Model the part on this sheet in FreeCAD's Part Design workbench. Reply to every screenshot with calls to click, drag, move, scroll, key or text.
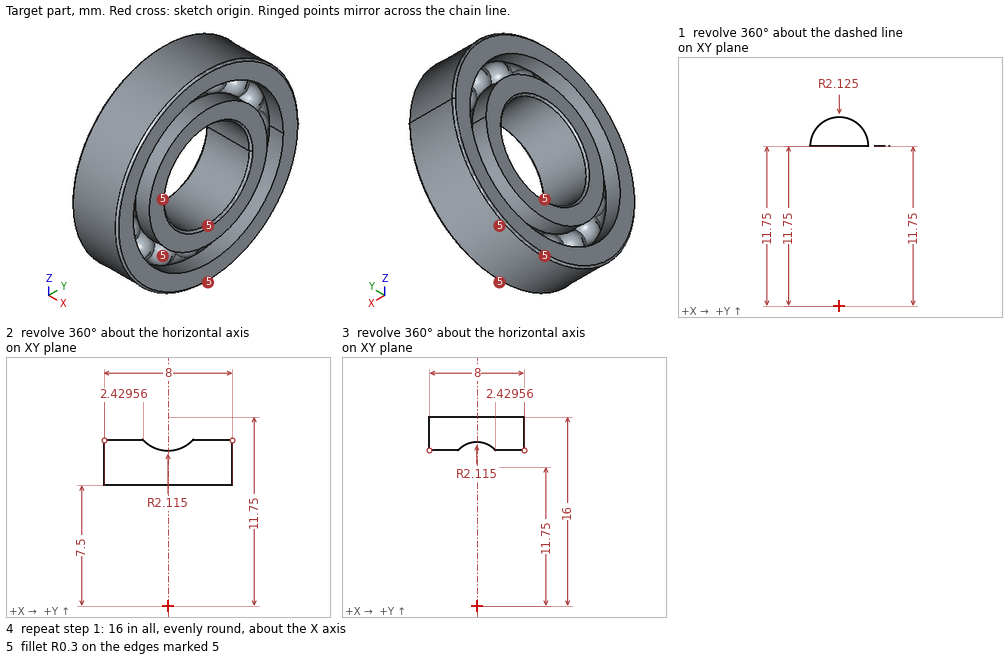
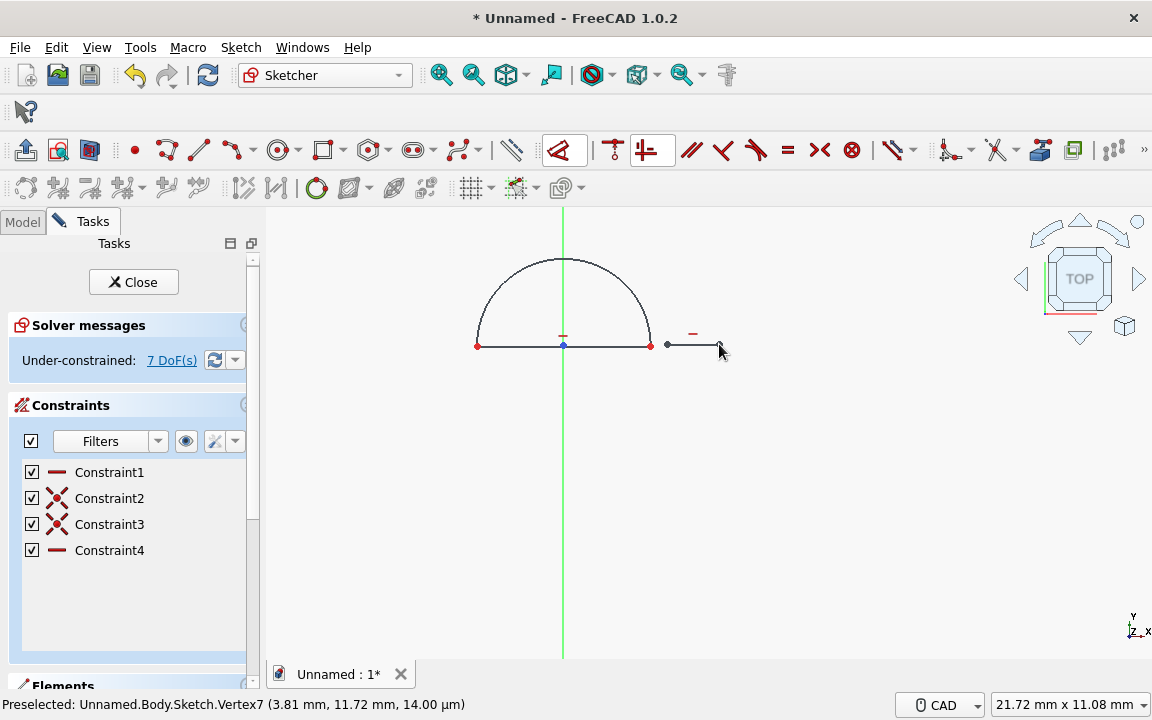
click(683, 345)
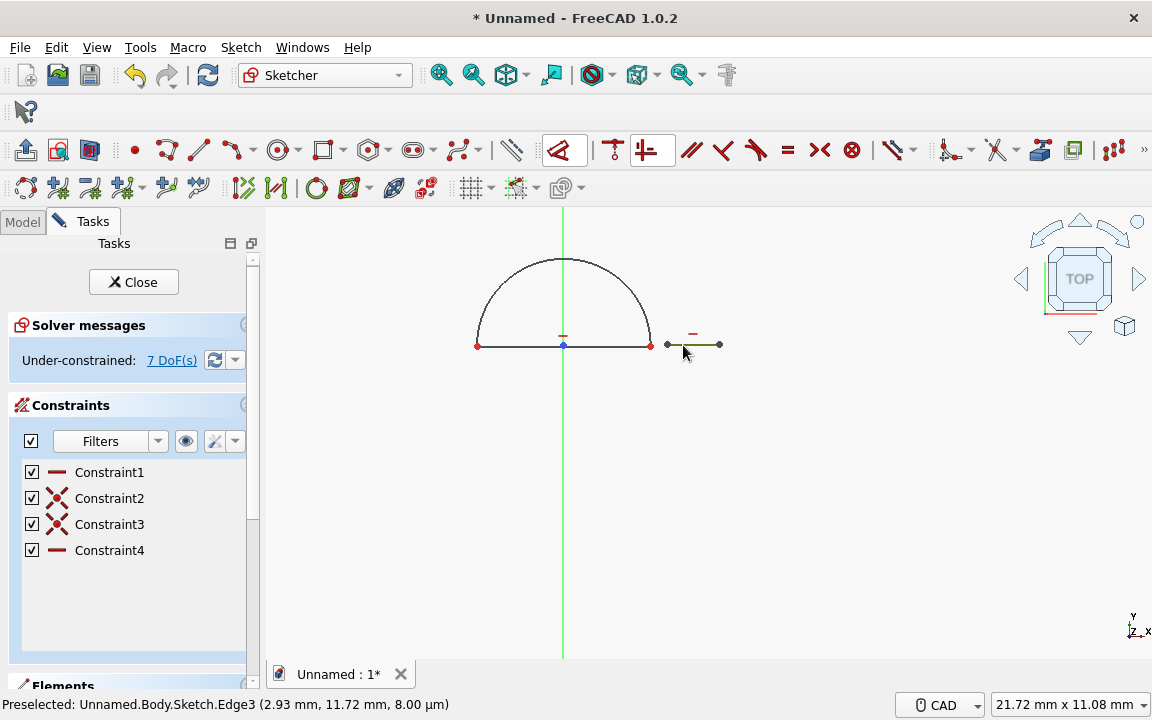
click(512, 150)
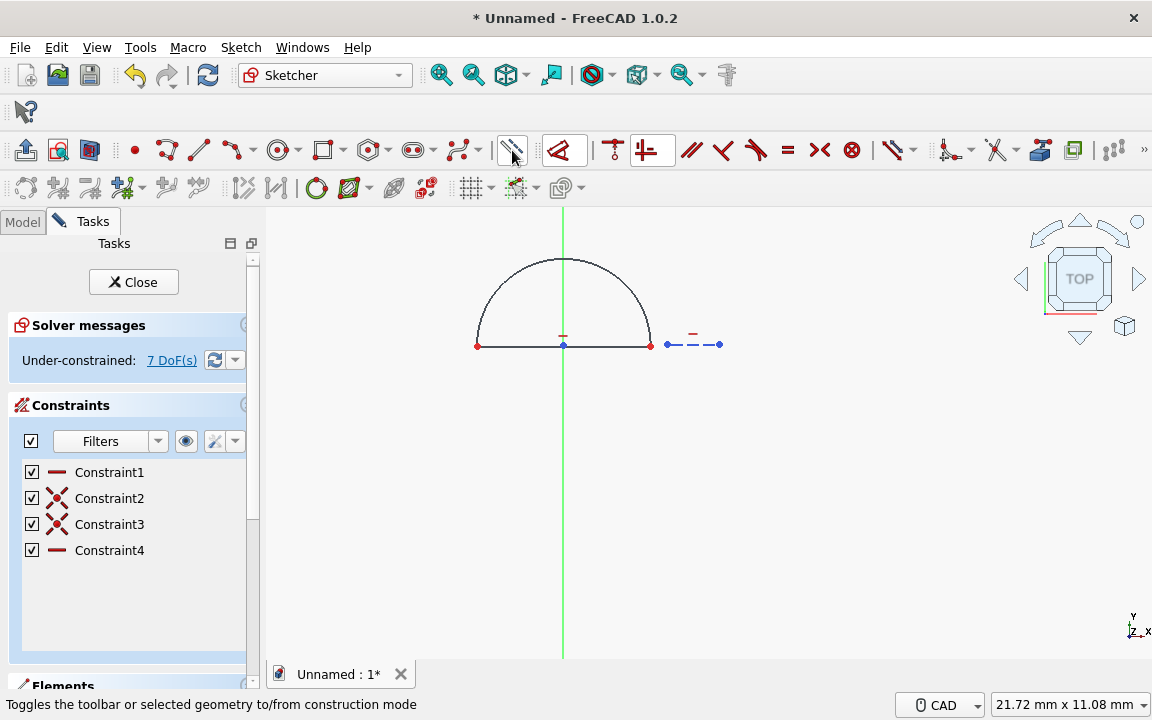
click(564, 346)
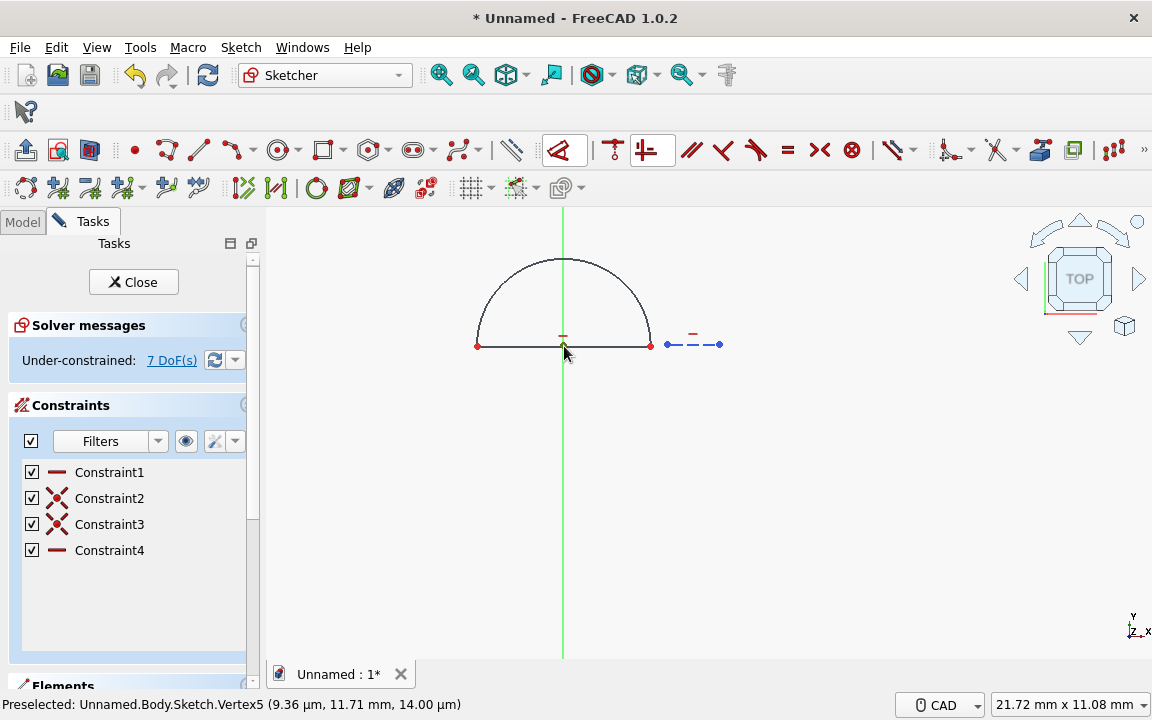
click(563, 603)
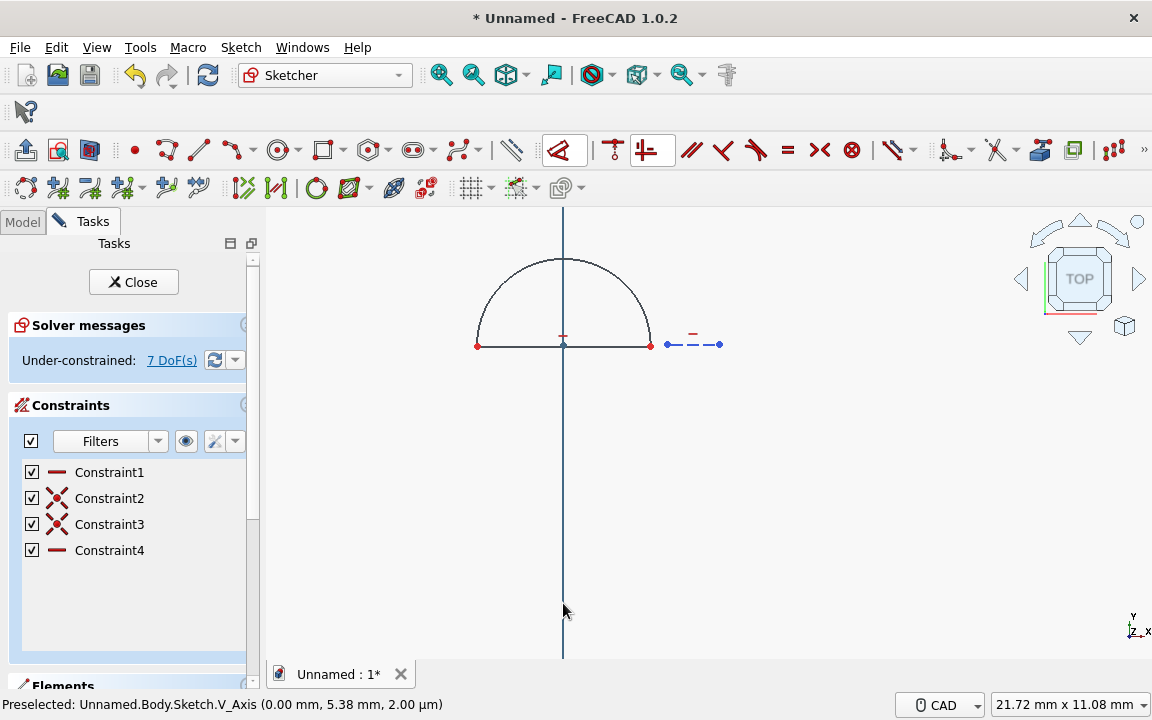
click(614, 150)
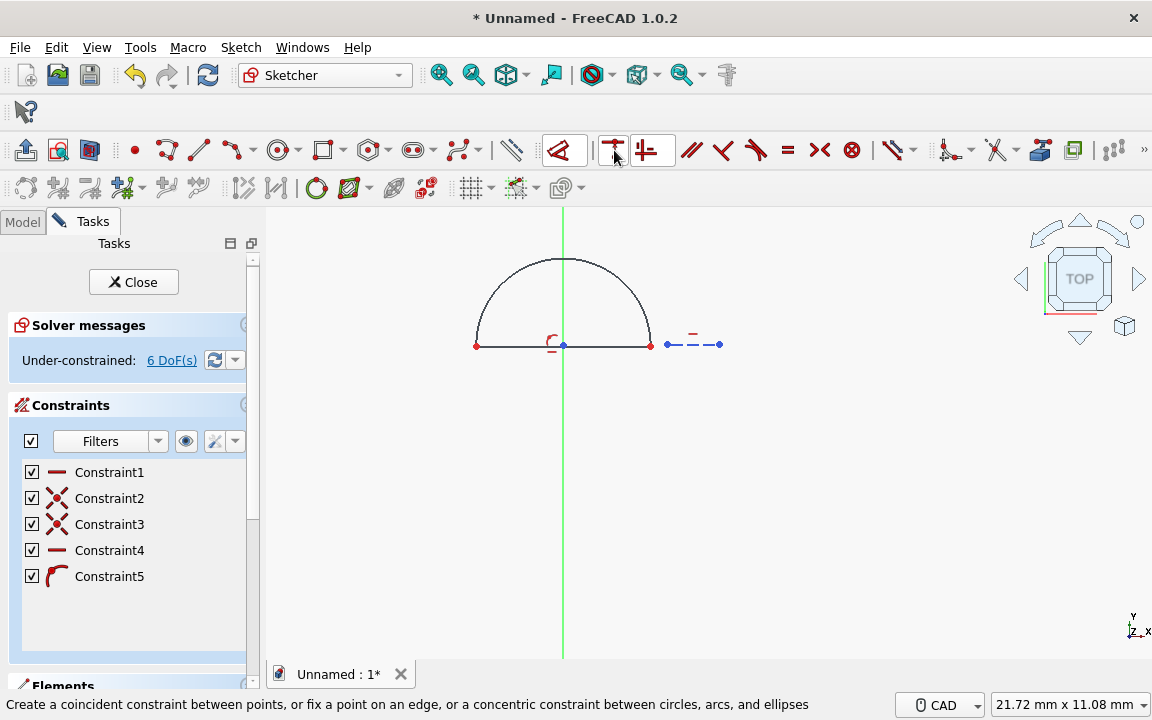
click(558, 150)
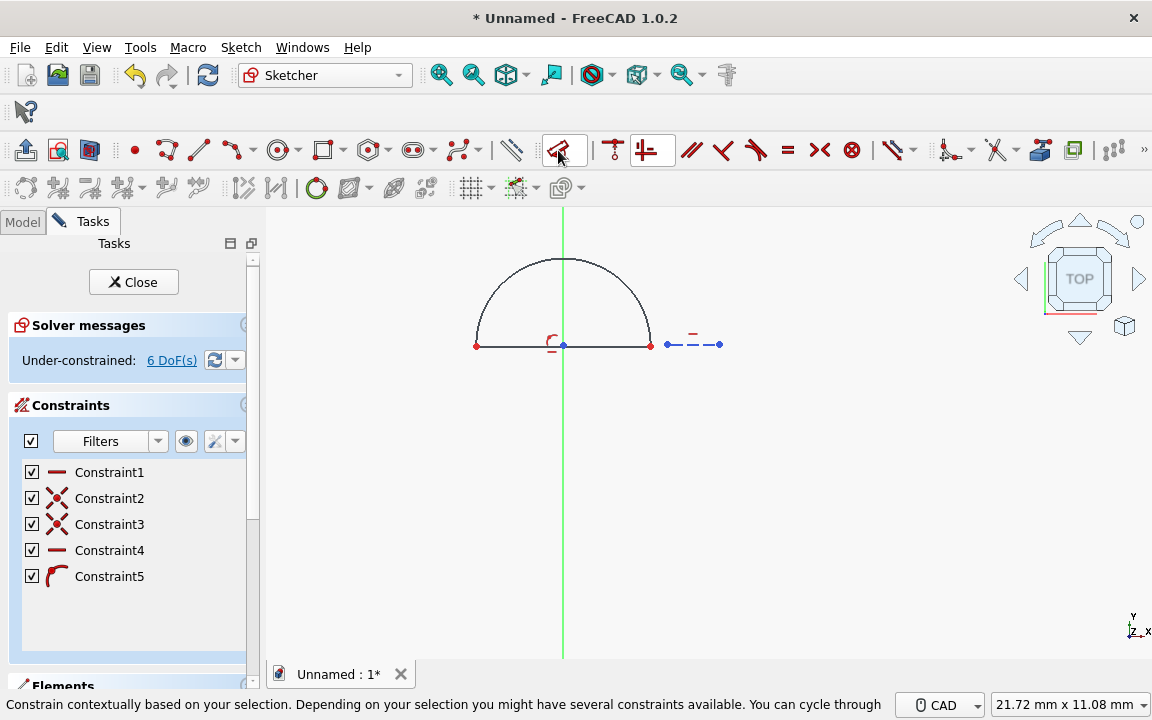
click(615, 275)
click(634, 249)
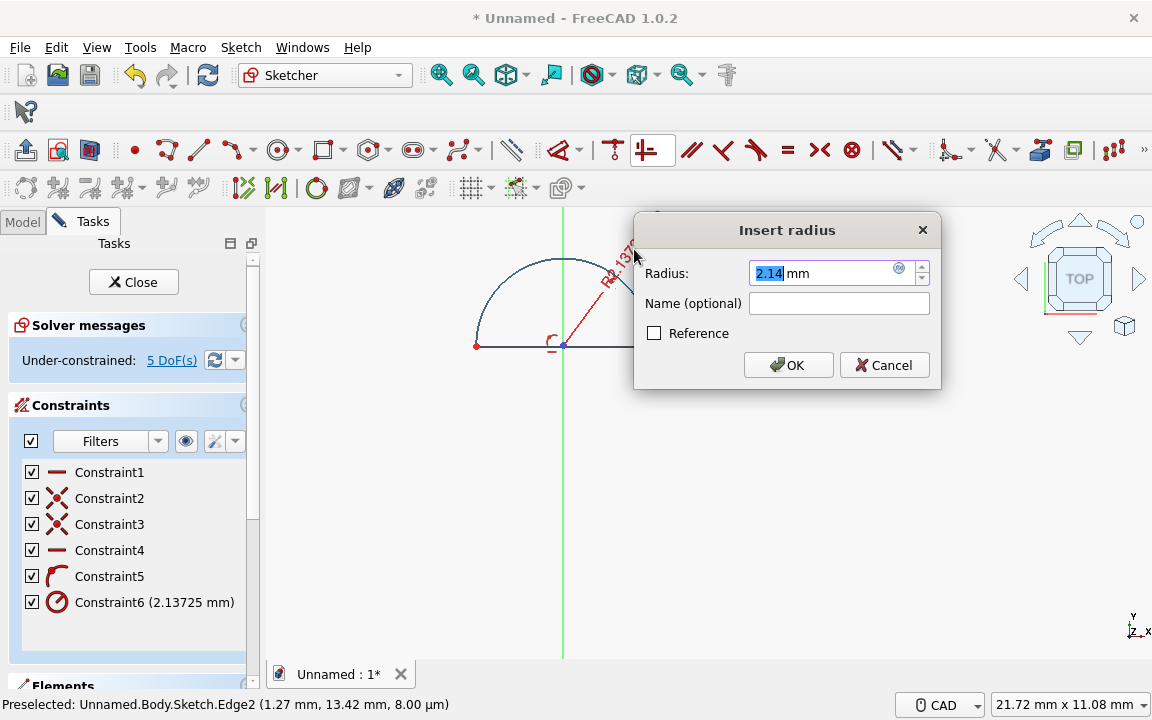
text(2.125)
key(Return)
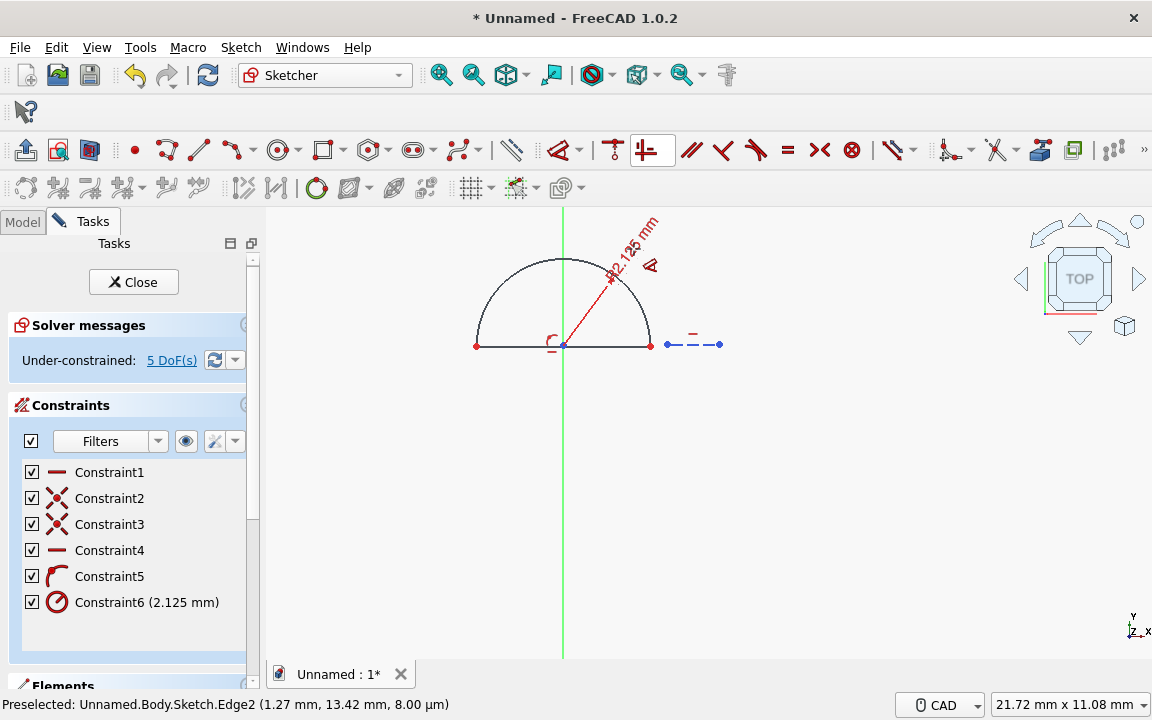
click(477, 347)
click(443, 489)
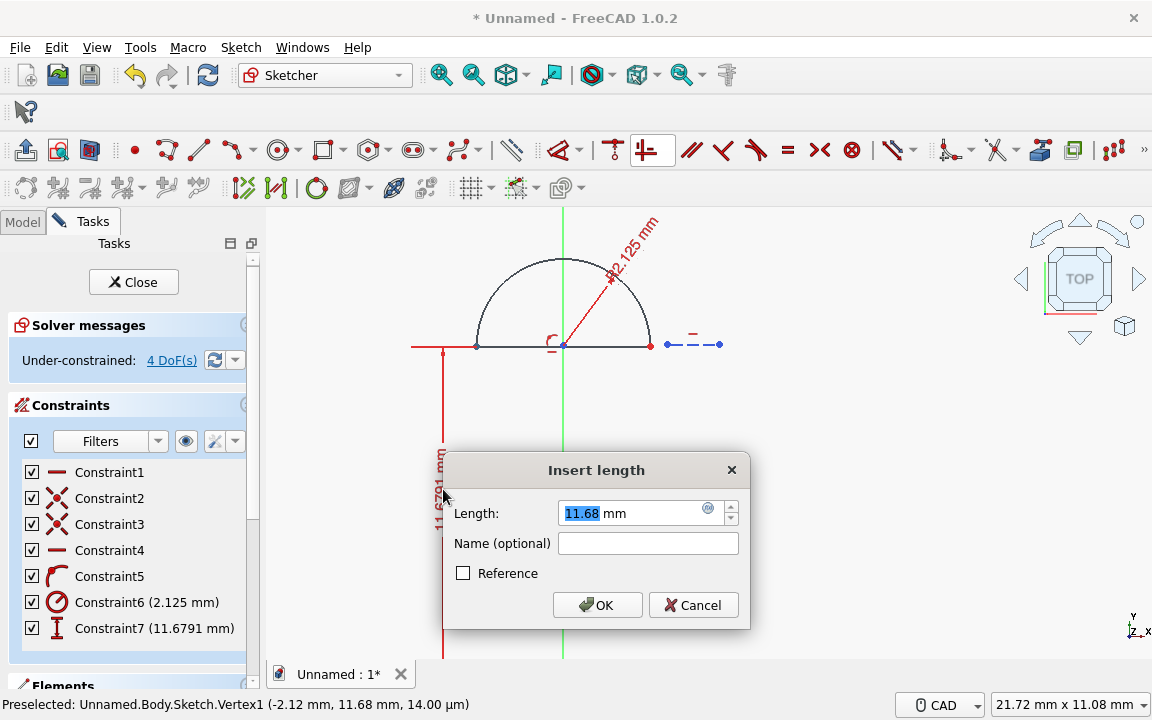
text(11.75)
key(Return)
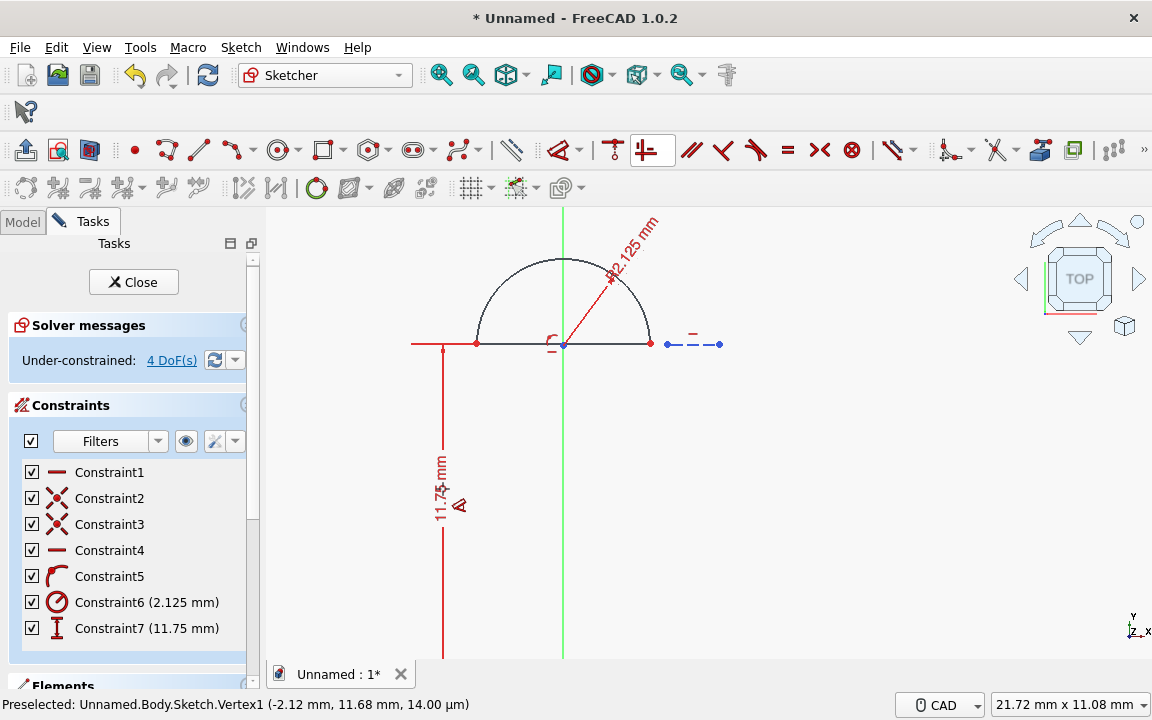
click(667, 345)
click(701, 488)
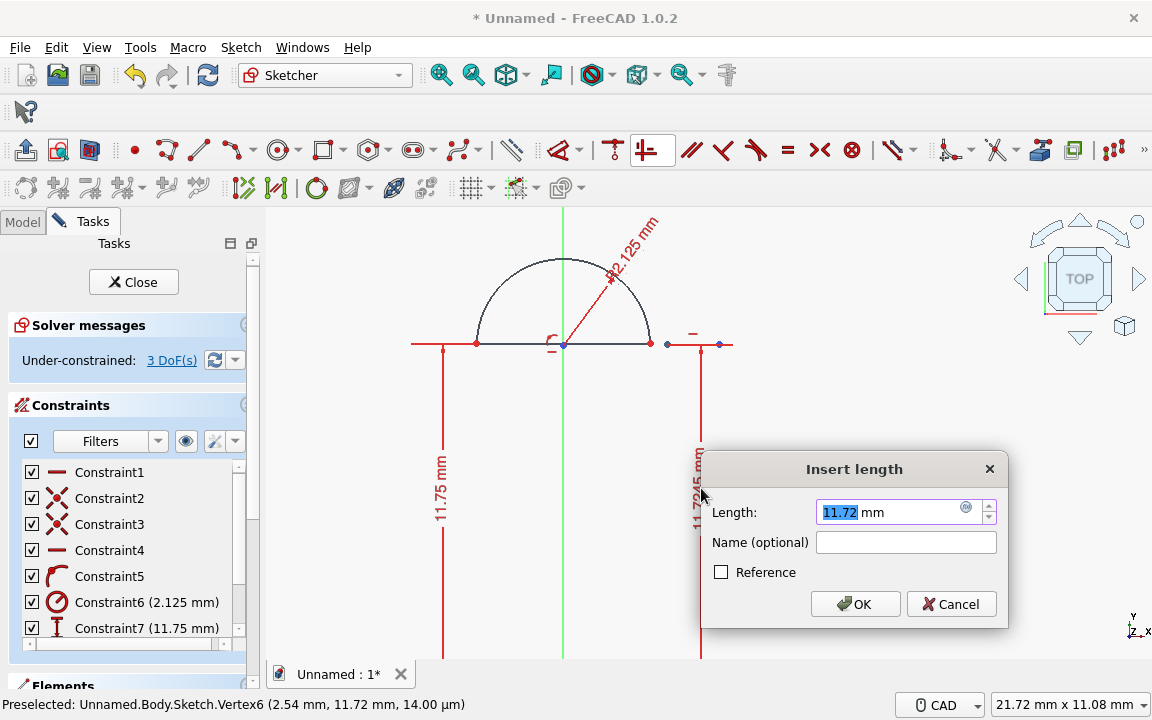
text(11.75)
key(Return)